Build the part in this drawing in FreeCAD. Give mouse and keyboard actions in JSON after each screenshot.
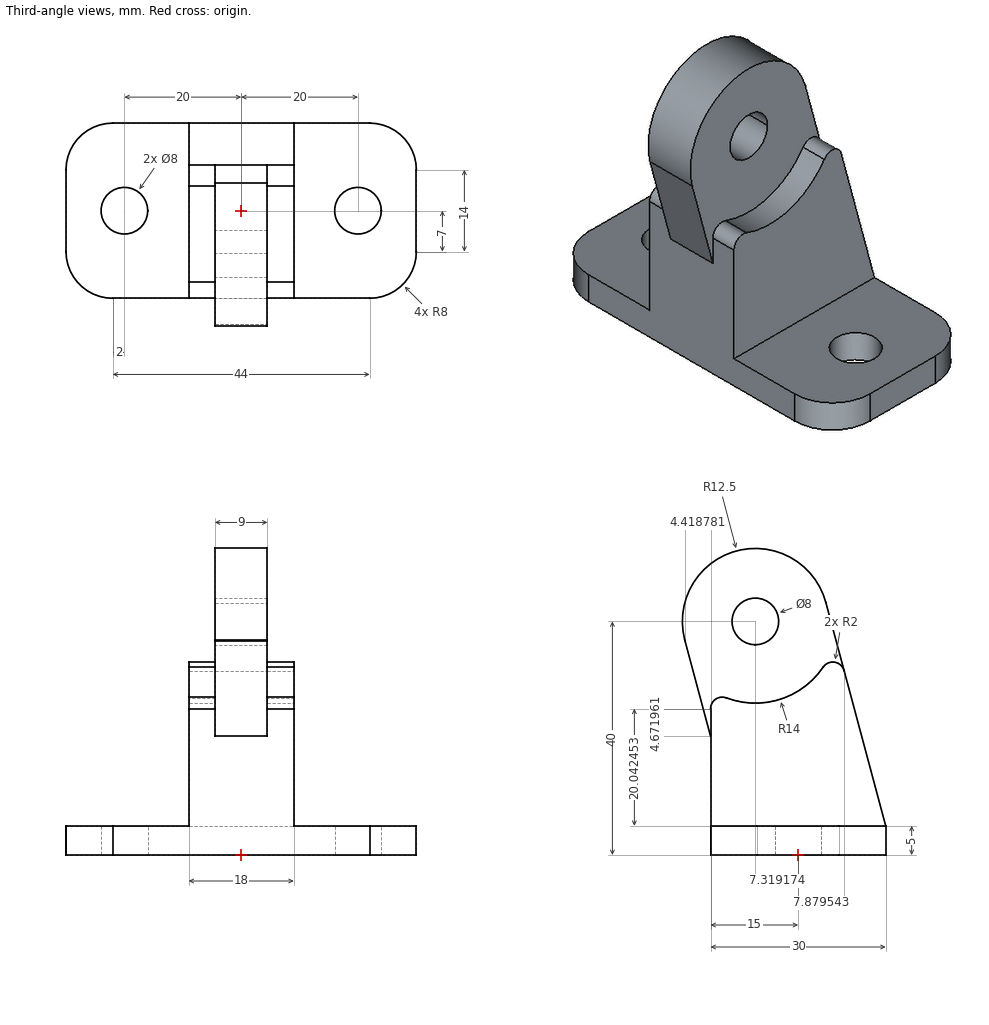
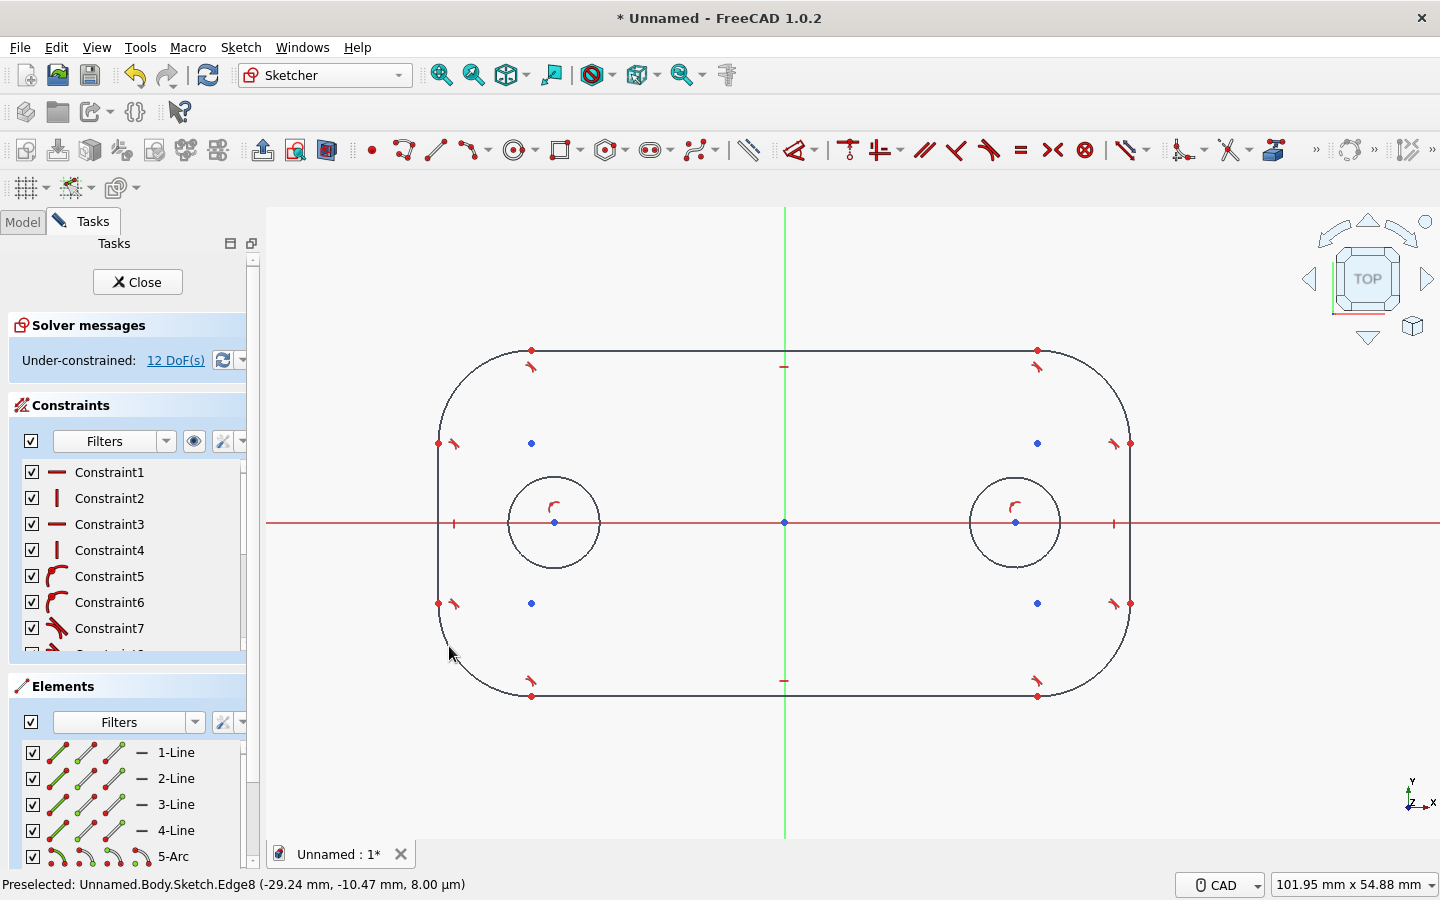
{"action": "left_click", "coordinate": [1080, 686]}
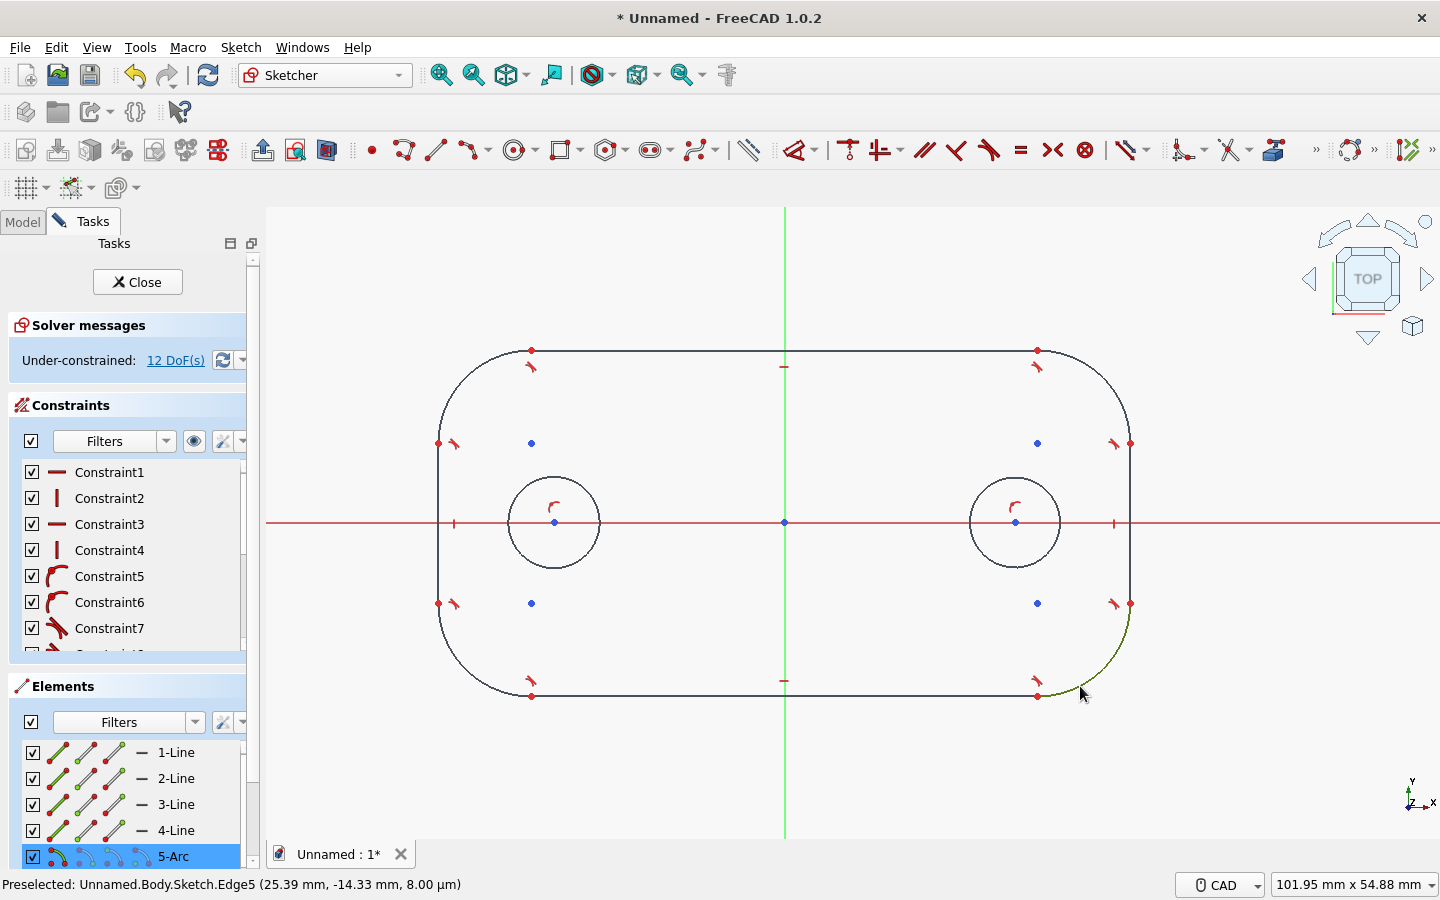
{"action": "left_click", "coordinate": [1120, 401]}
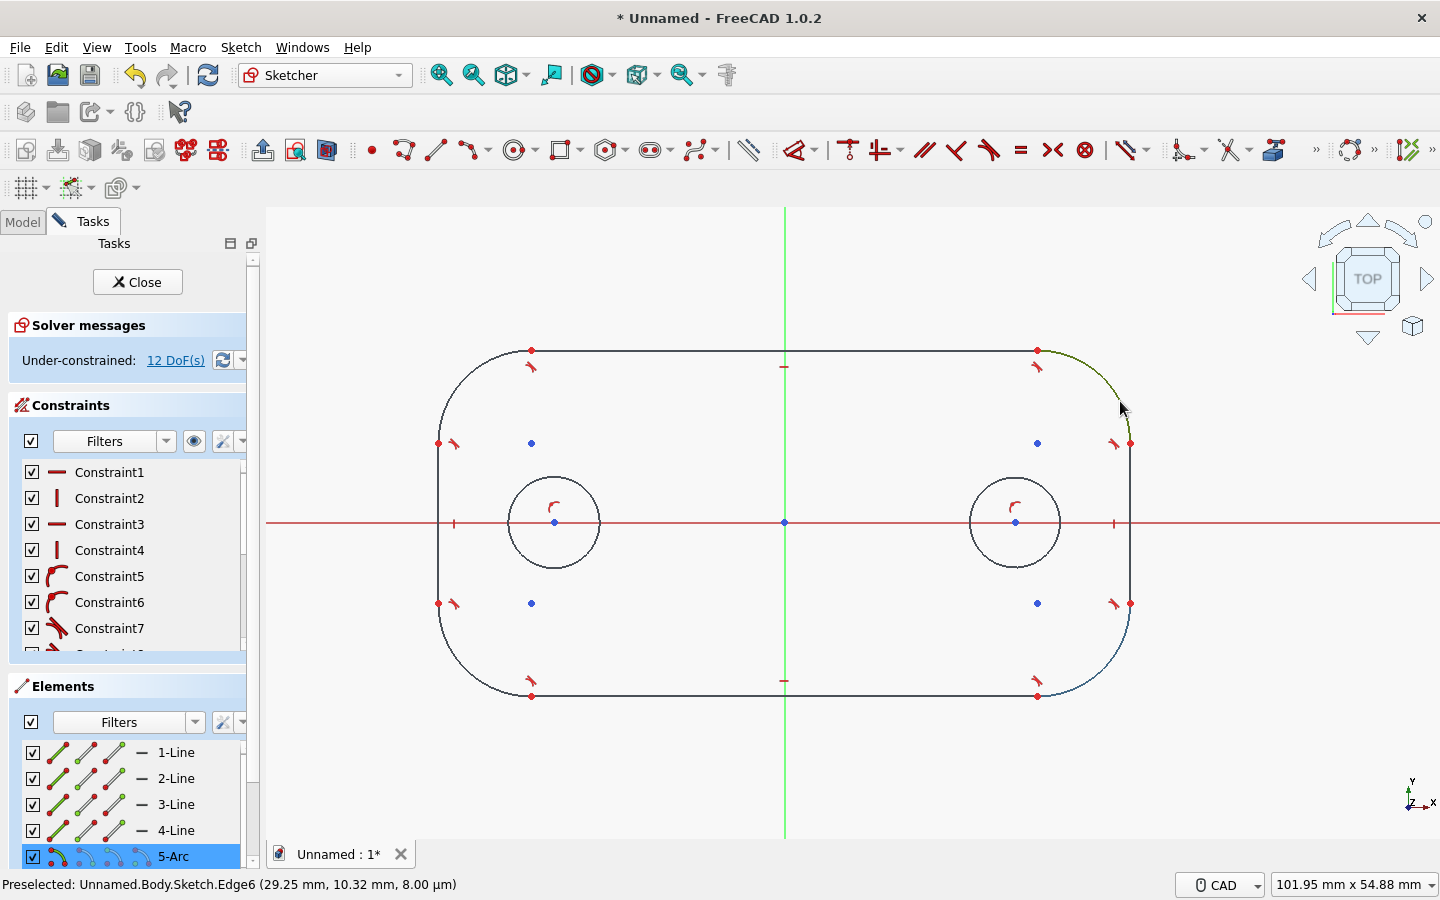
{"action": "left_click", "coordinate": [489, 361]}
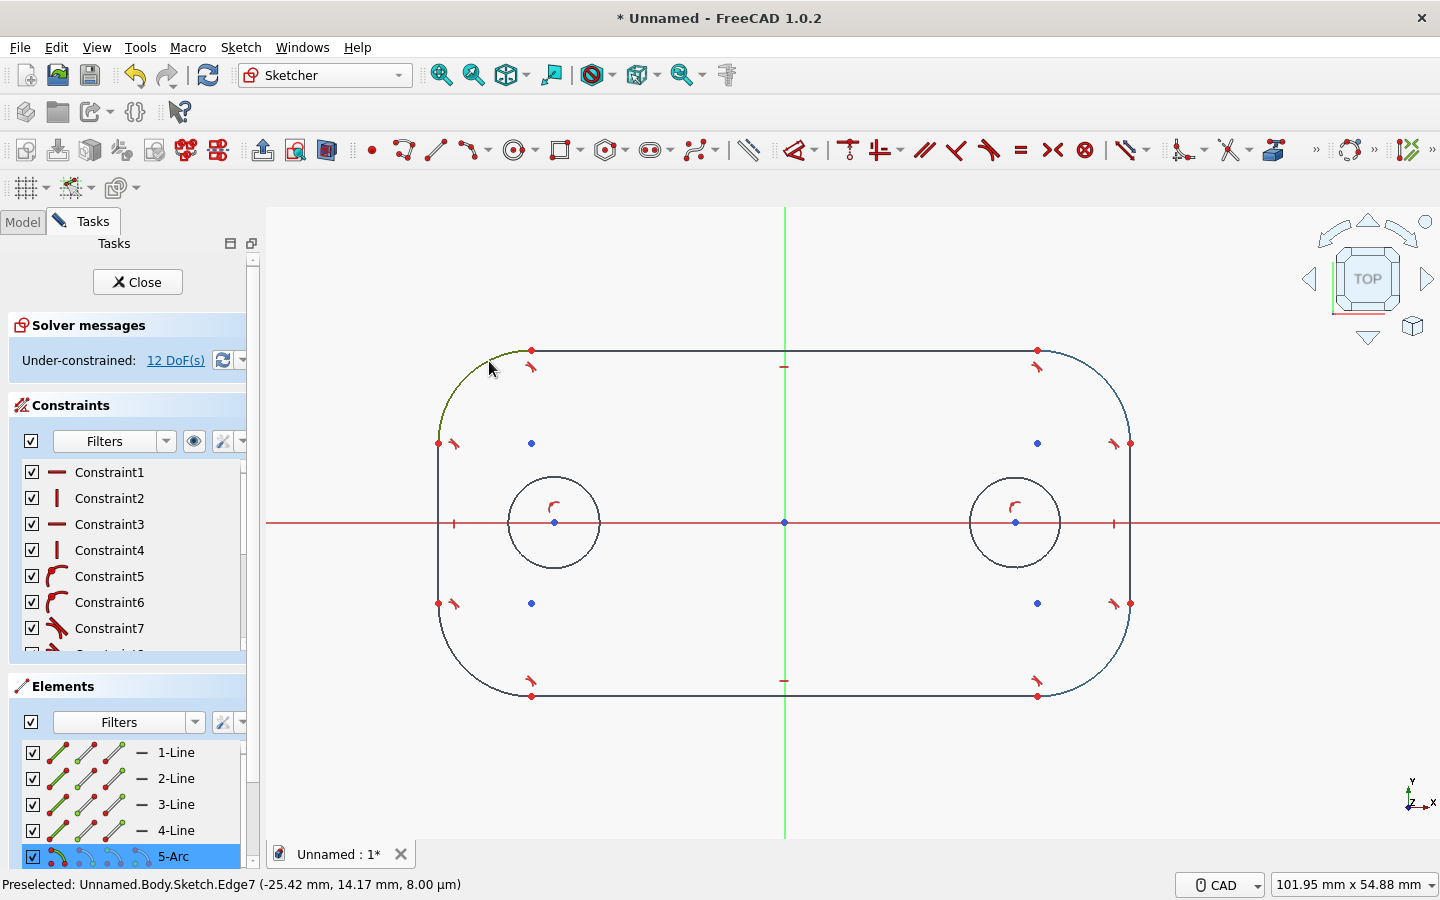
{"action": "left_click", "coordinate": [449, 646]}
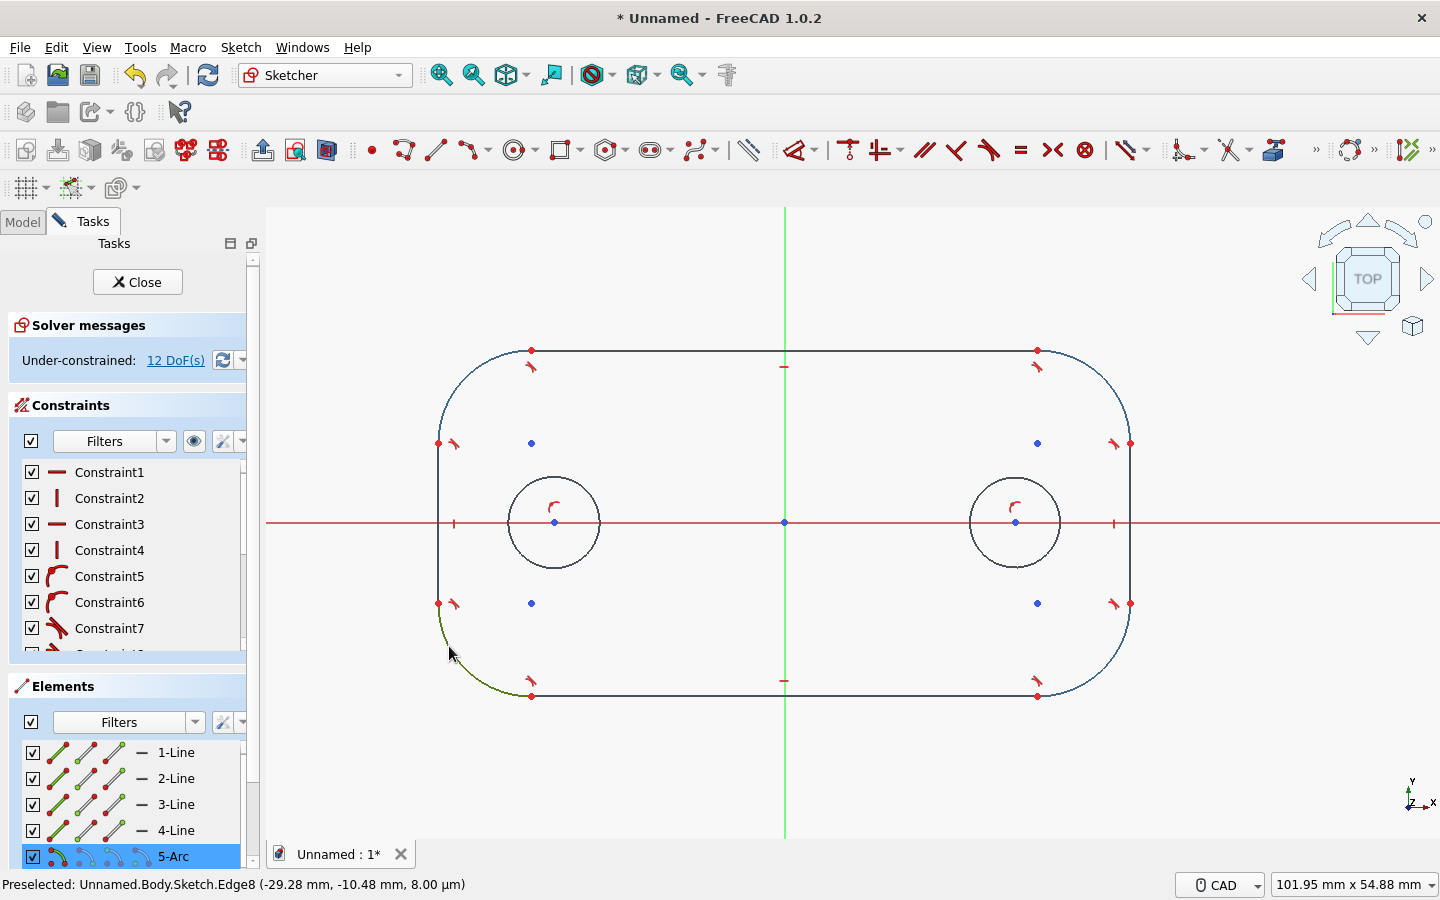
{"action": "key", "text": "e"}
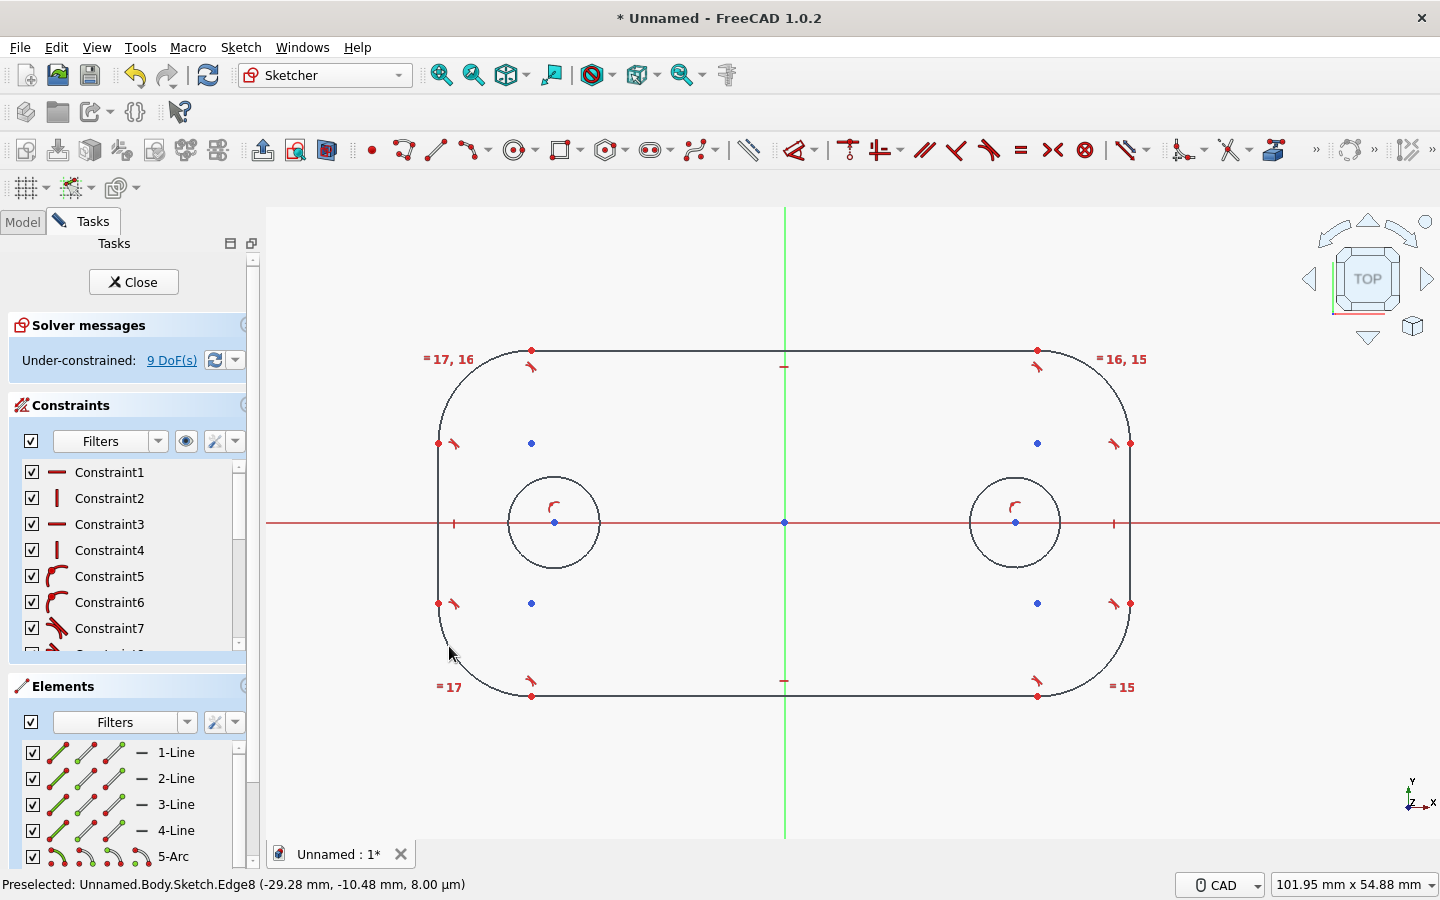
{"action": "left_click", "coordinate": [586, 490]}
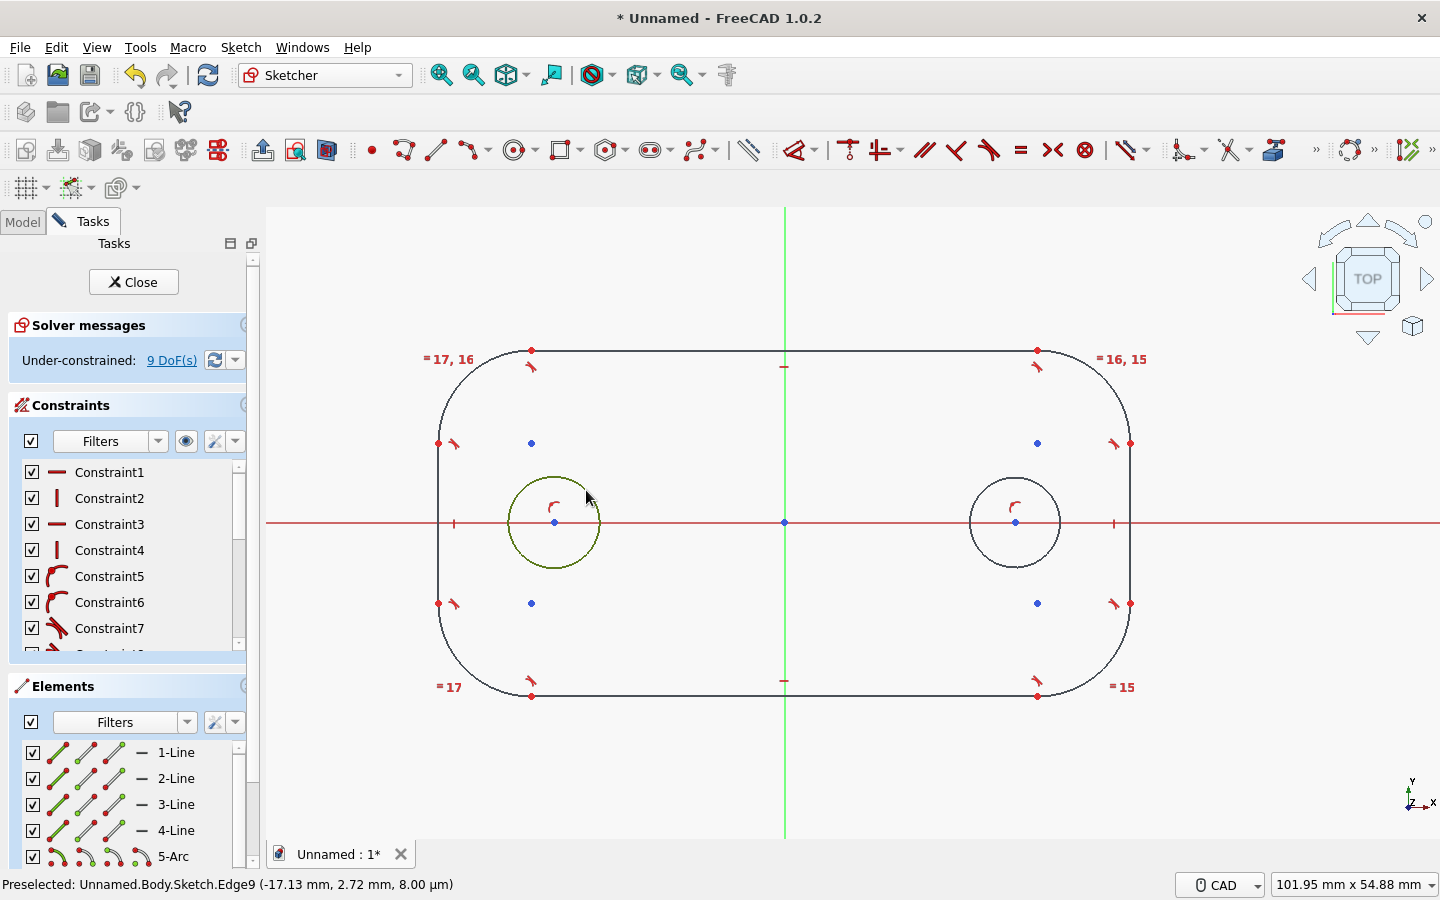
{"action": "left_click", "coordinate": [1047, 491]}